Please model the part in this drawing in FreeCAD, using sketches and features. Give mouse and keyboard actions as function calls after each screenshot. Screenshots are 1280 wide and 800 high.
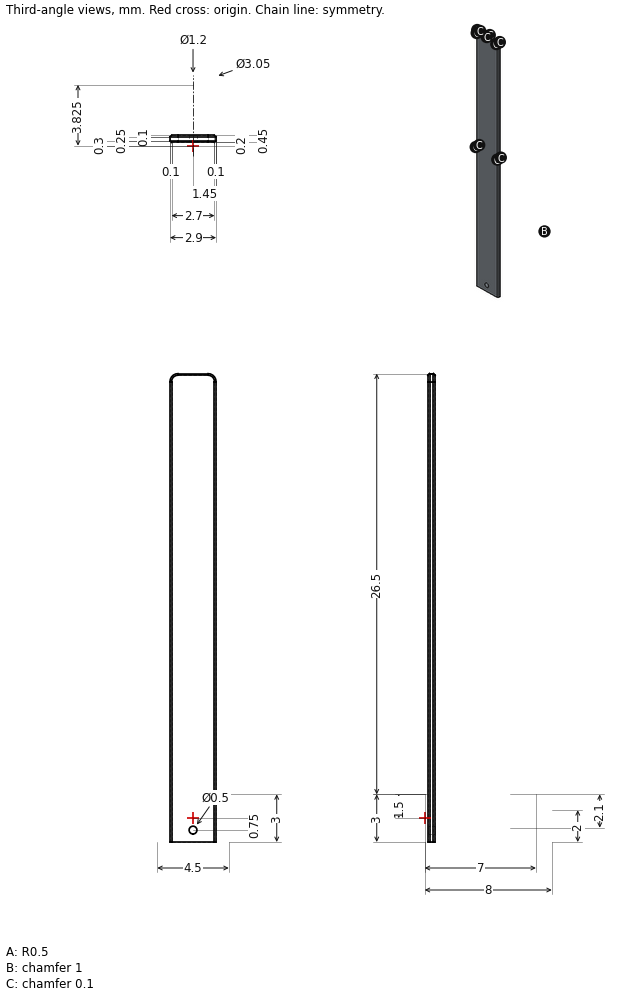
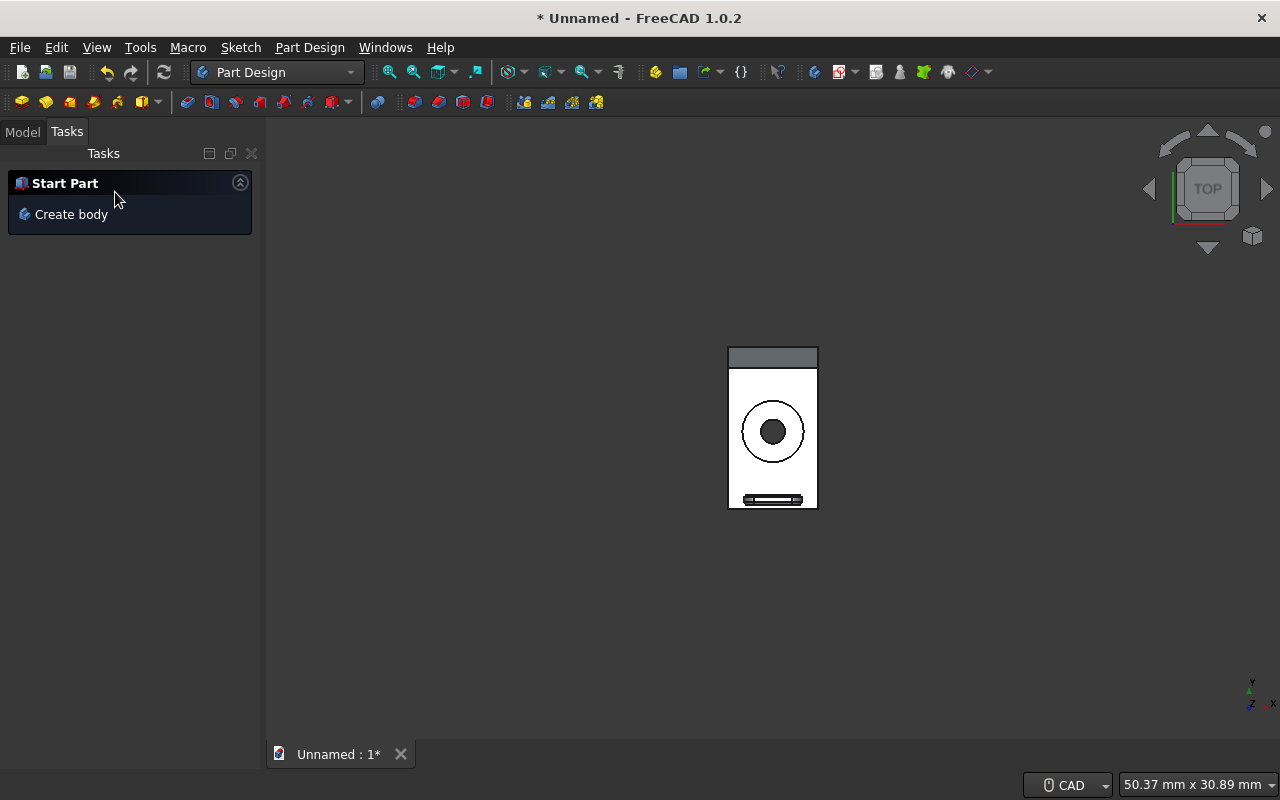
click(390, 72)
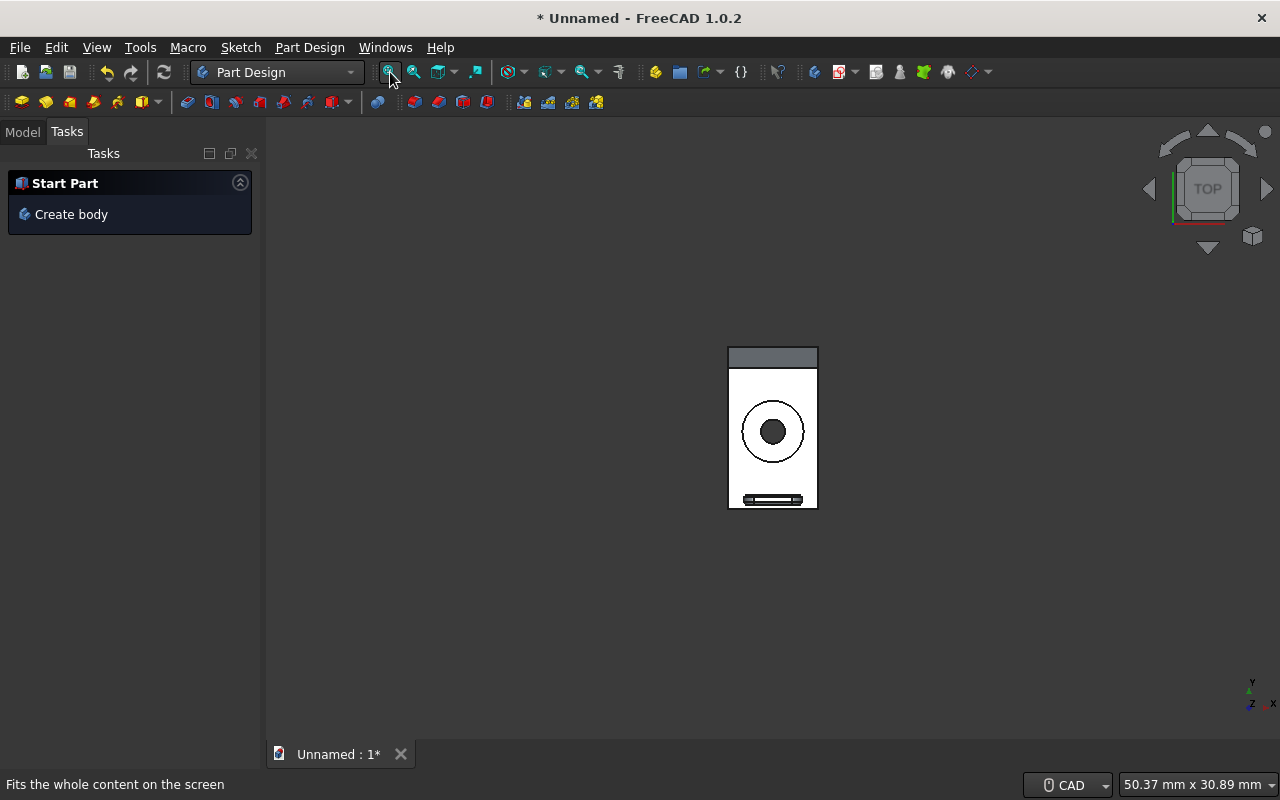
key(0)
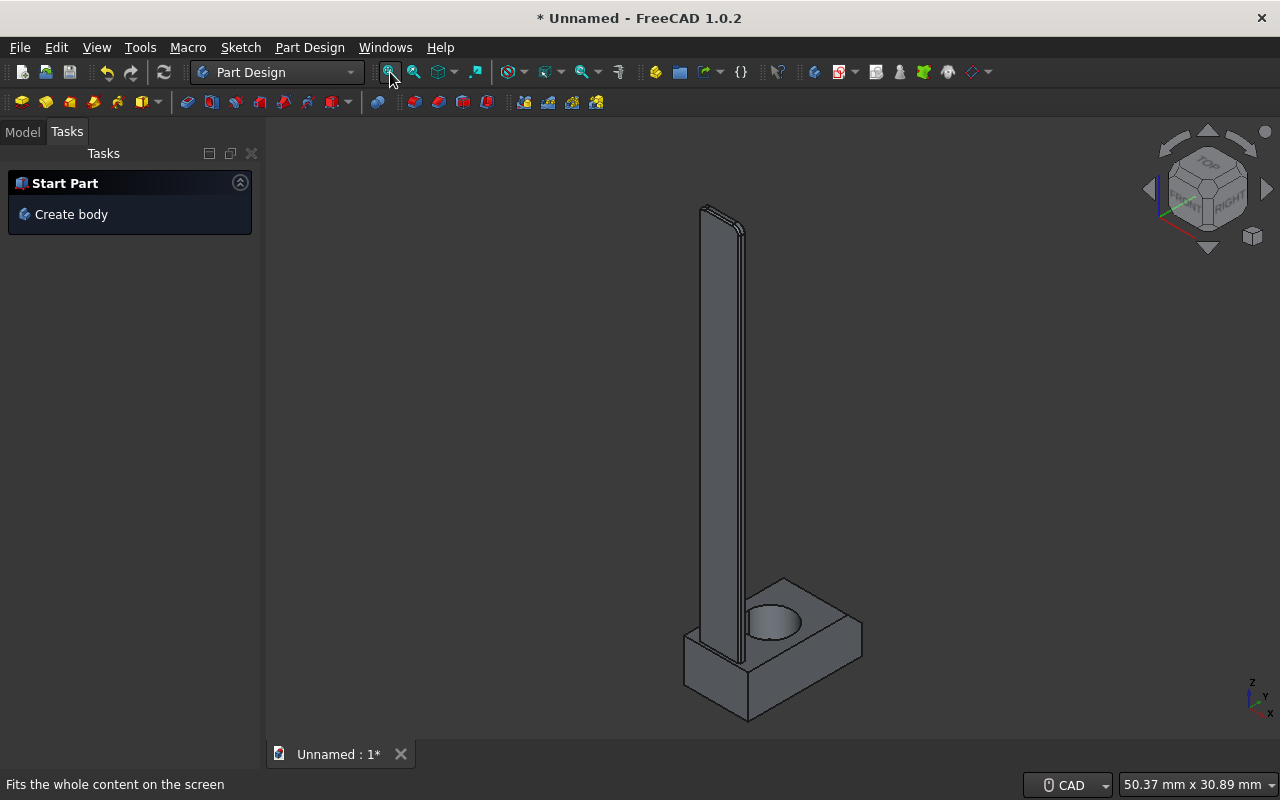
click(838, 645)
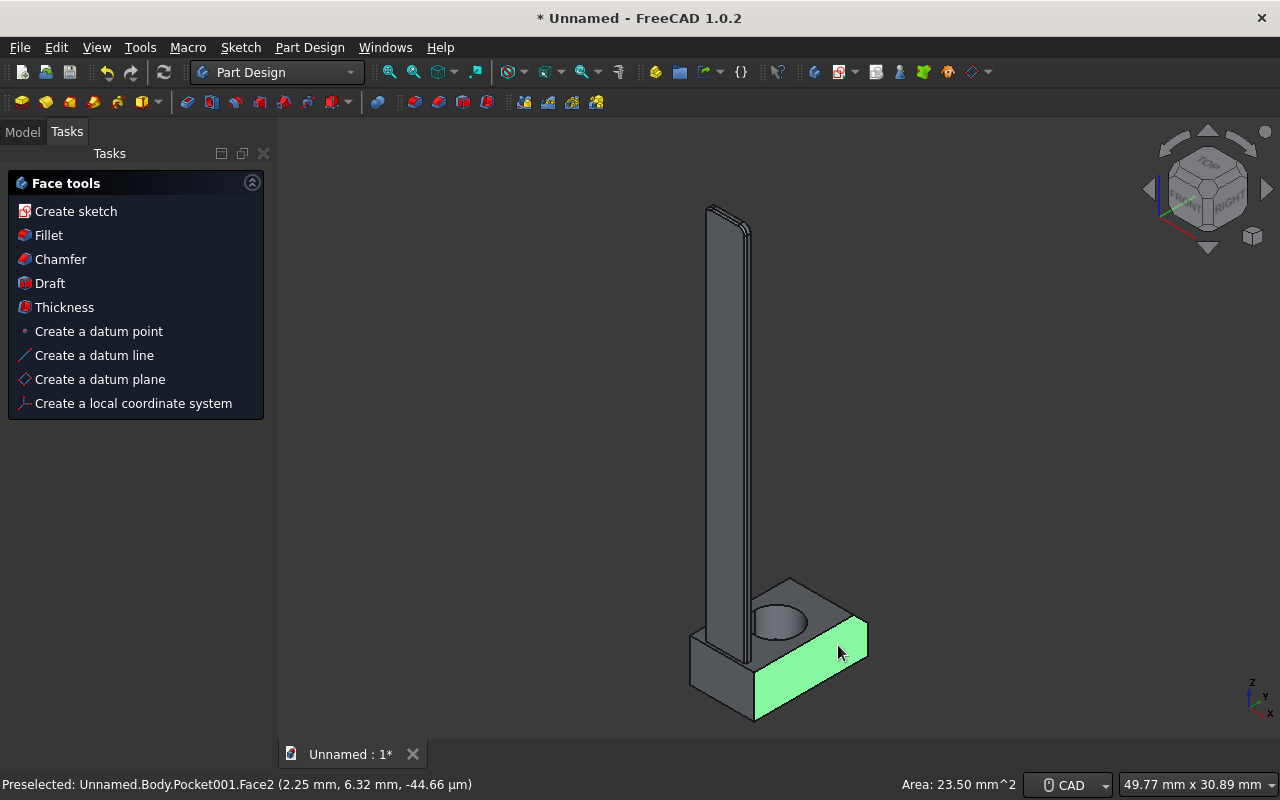
click(840, 72)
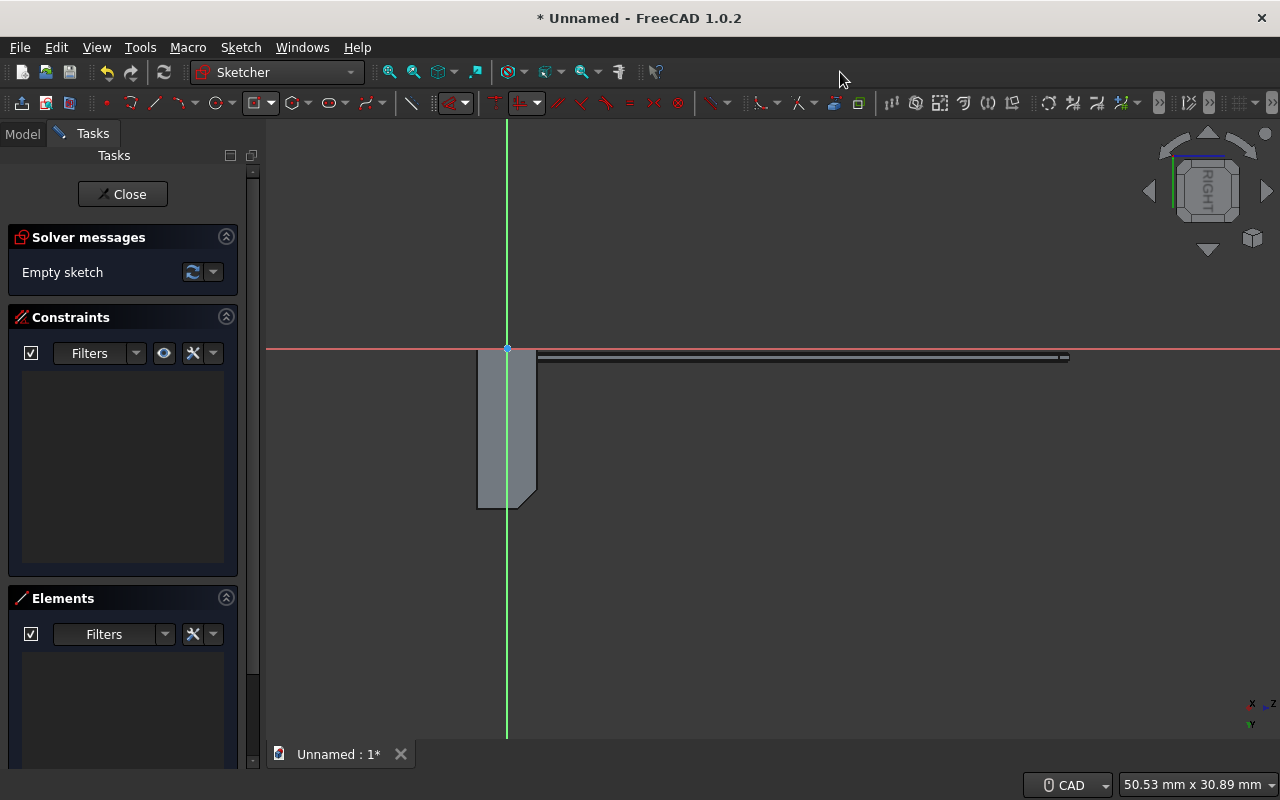
scroll(392, 429, up, 5)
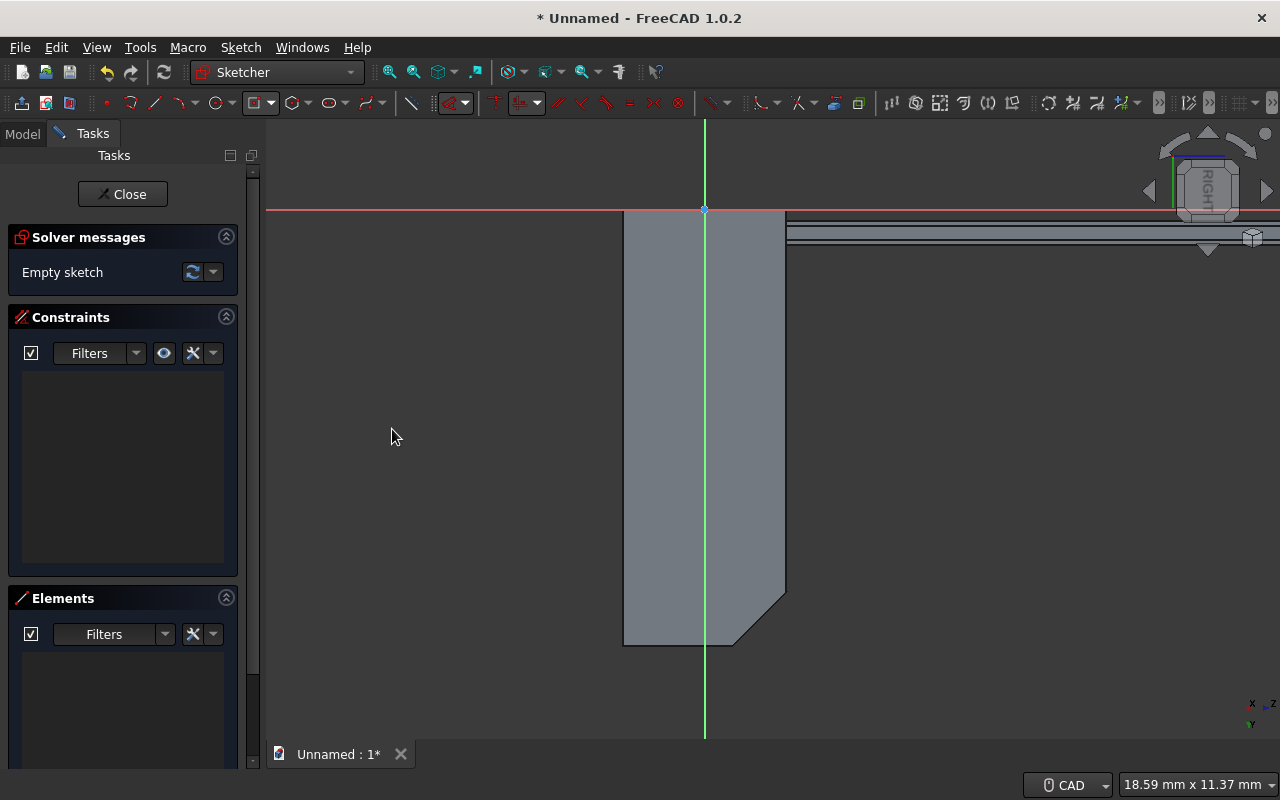
click(132, 104)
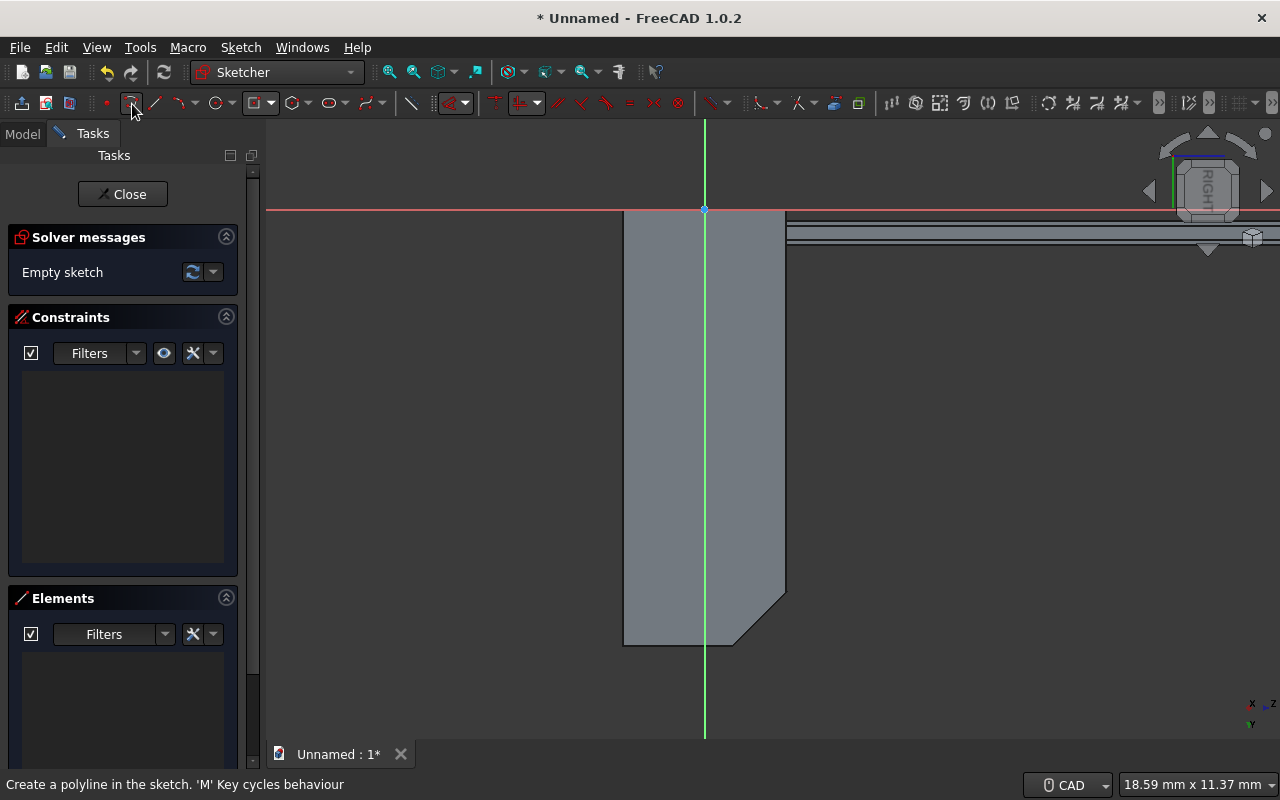
click(786, 210)
click(623, 219)
click(623, 646)
click(732, 646)
click(786, 592)
click(786, 210)
key(Escape)
key(Escape)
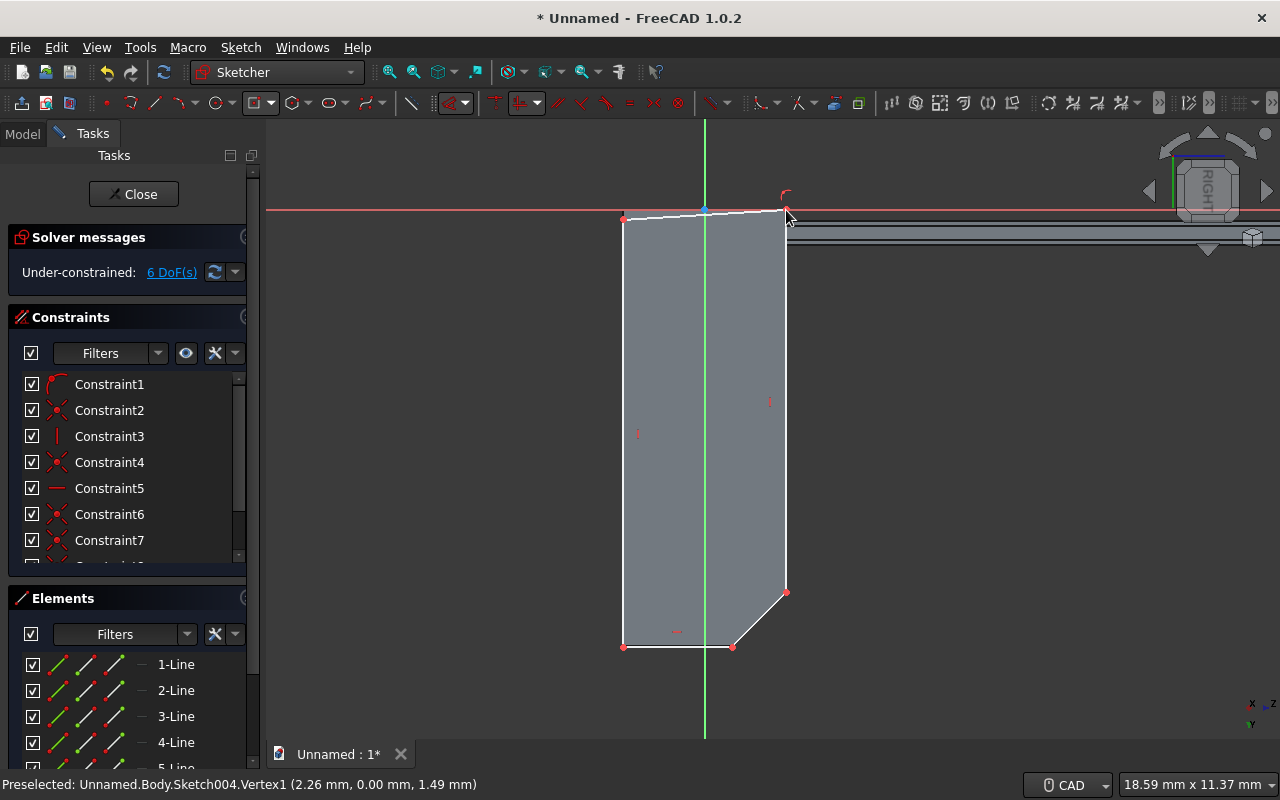
click(737, 213)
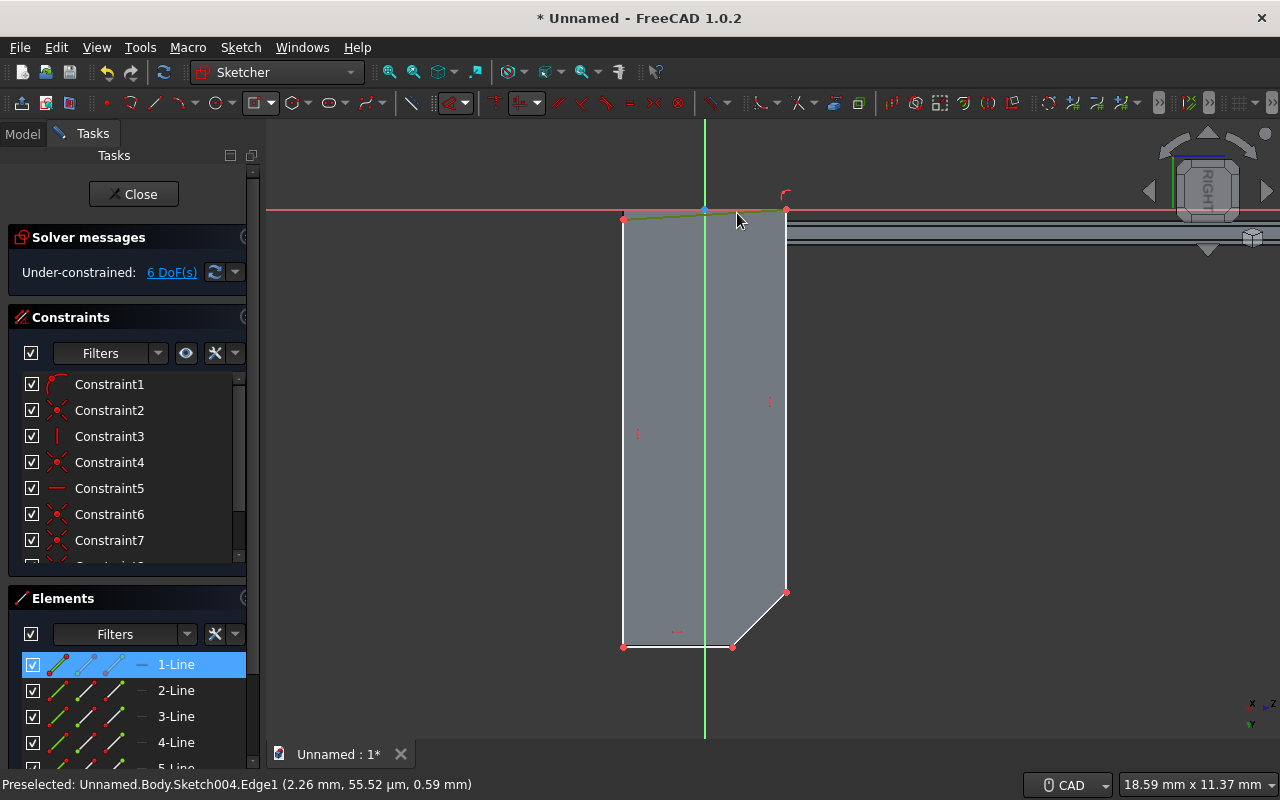
key(h)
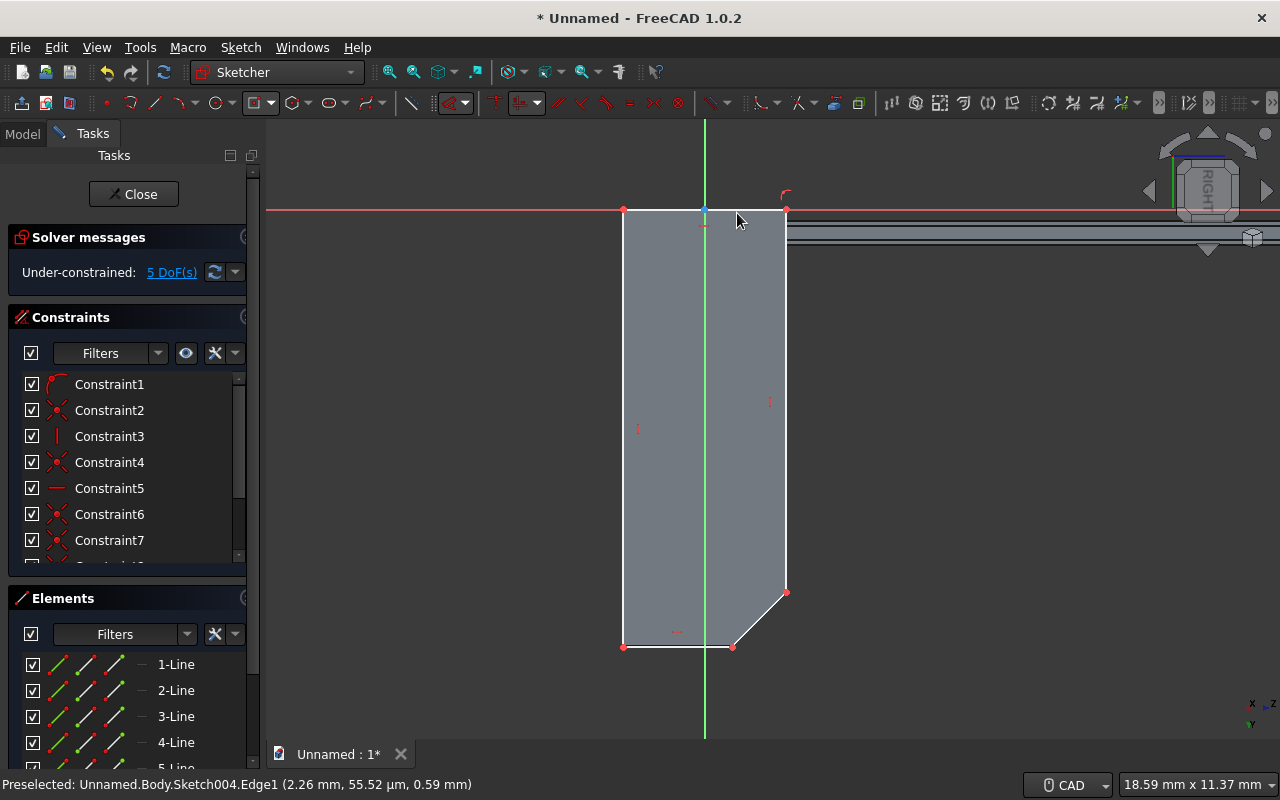
click(450, 104)